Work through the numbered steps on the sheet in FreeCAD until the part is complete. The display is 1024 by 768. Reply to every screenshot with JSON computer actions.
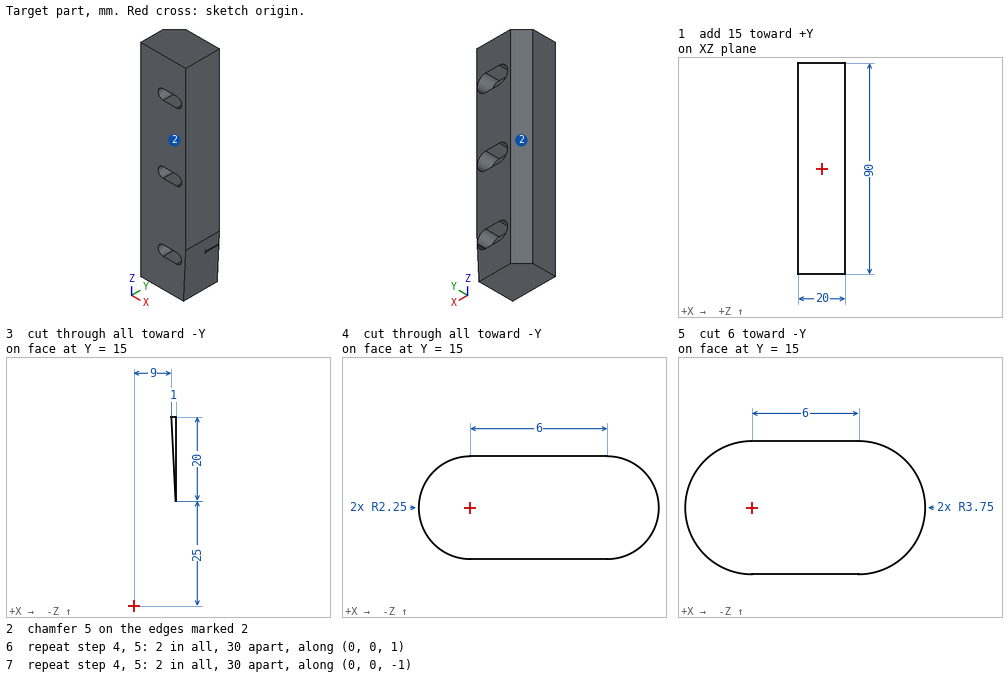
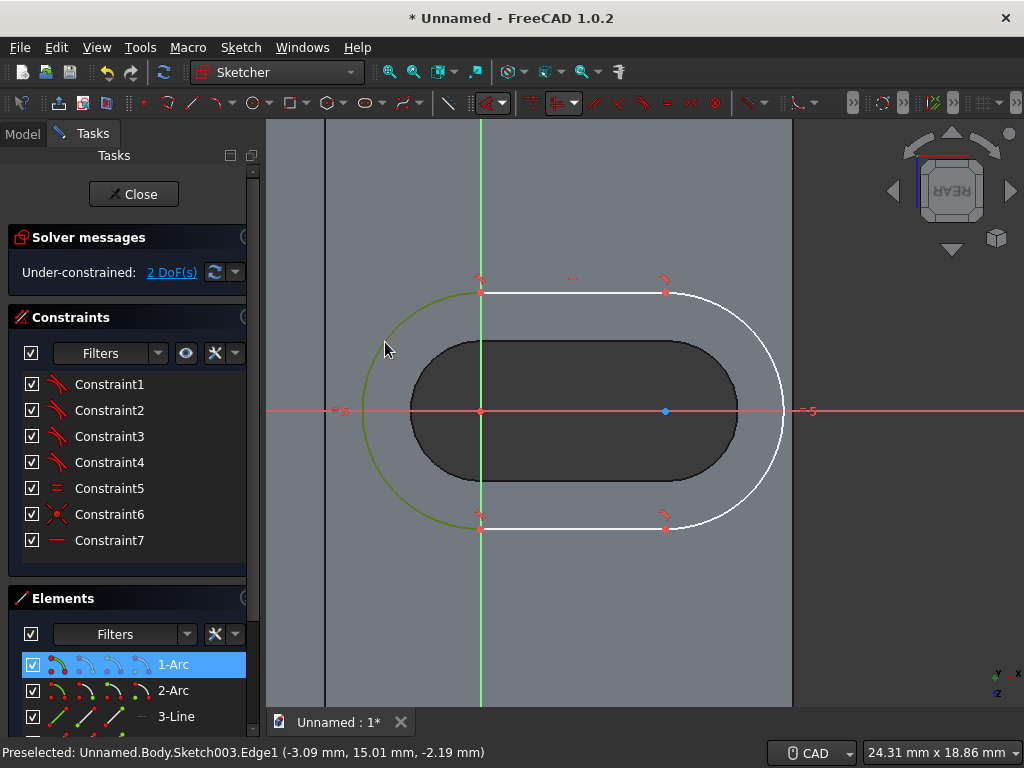
{"action": "left_click", "coordinate": [504, 104]}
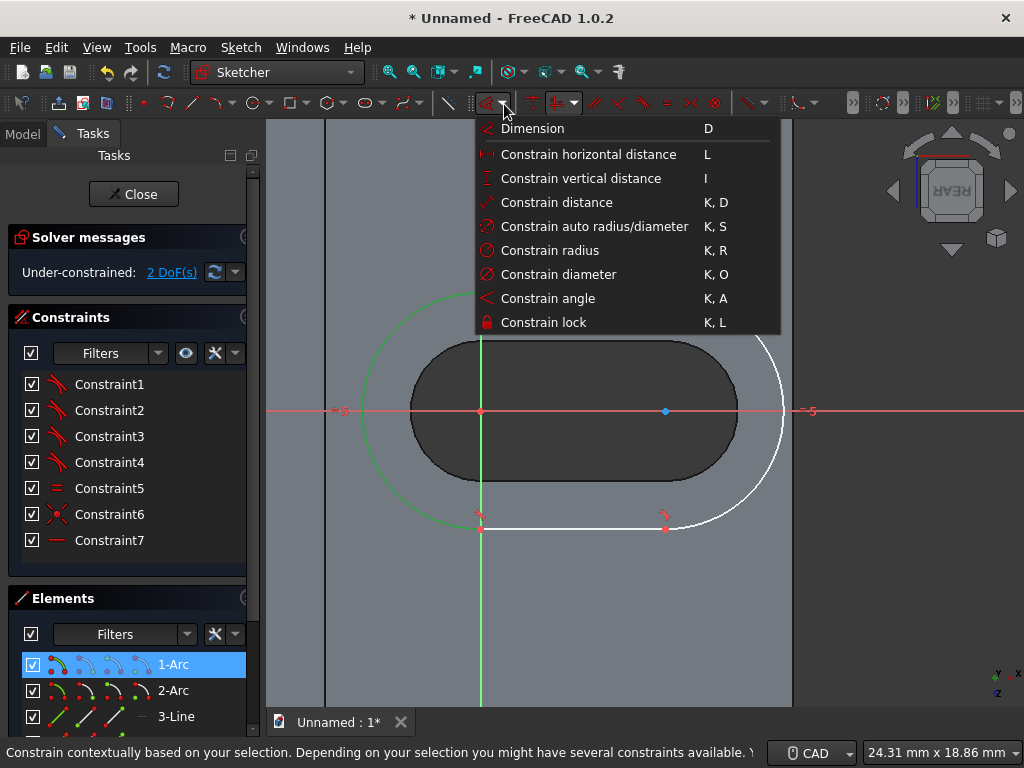
{"action": "left_click", "coordinate": [628, 250]}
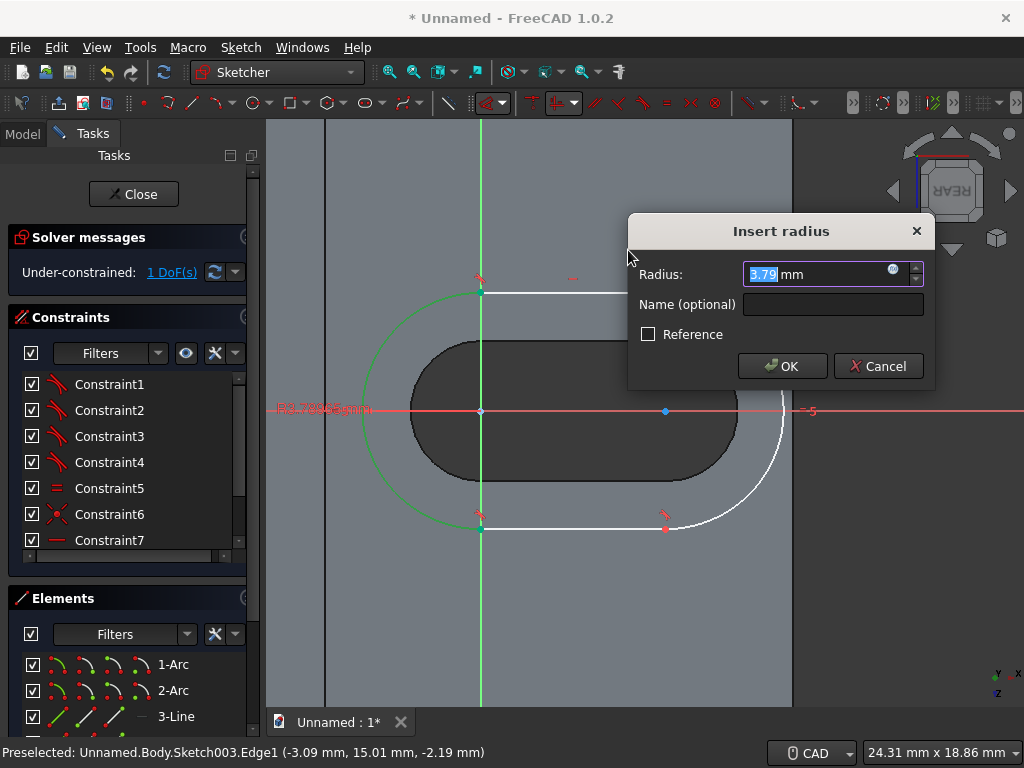
{"action": "type", "text": "3.75"}
{"action": "key", "text": "Return"}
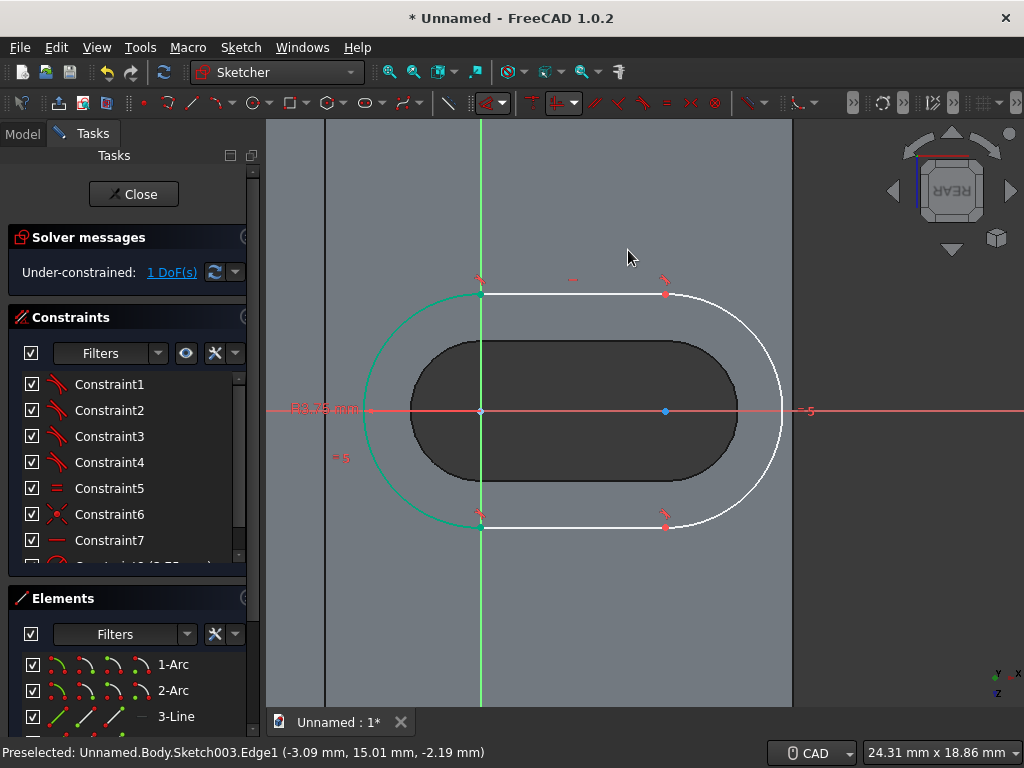
{"action": "left_click", "coordinate": [536, 294]}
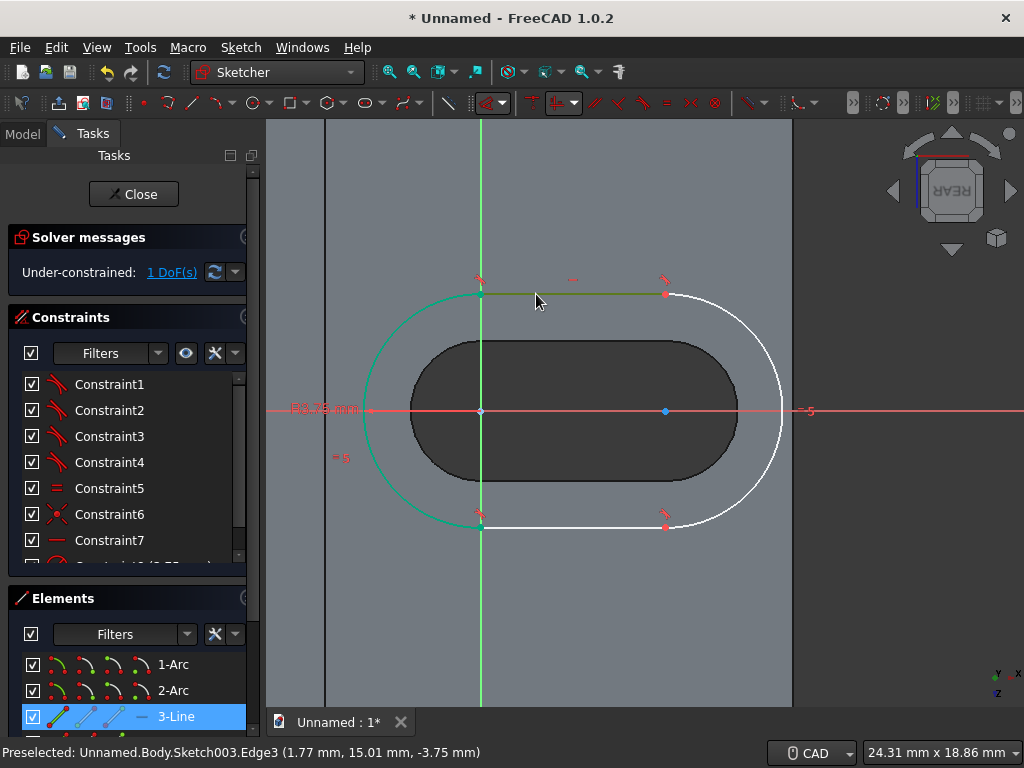
{"action": "left_click", "coordinate": [504, 104]}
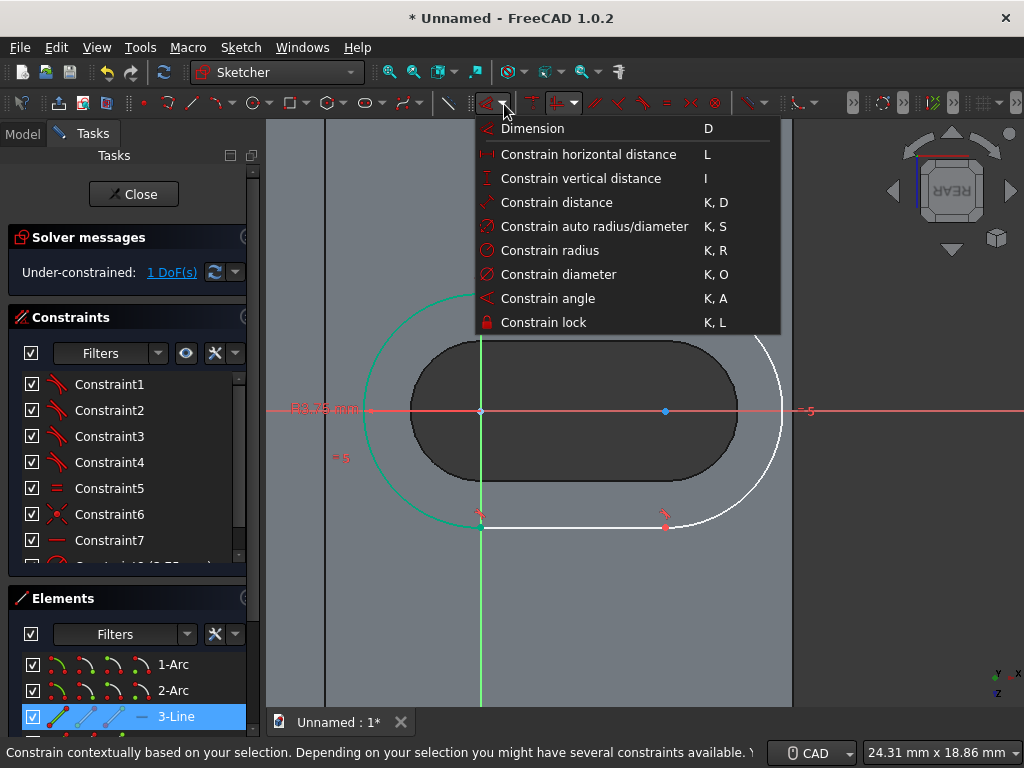
{"action": "left_click", "coordinate": [628, 154]}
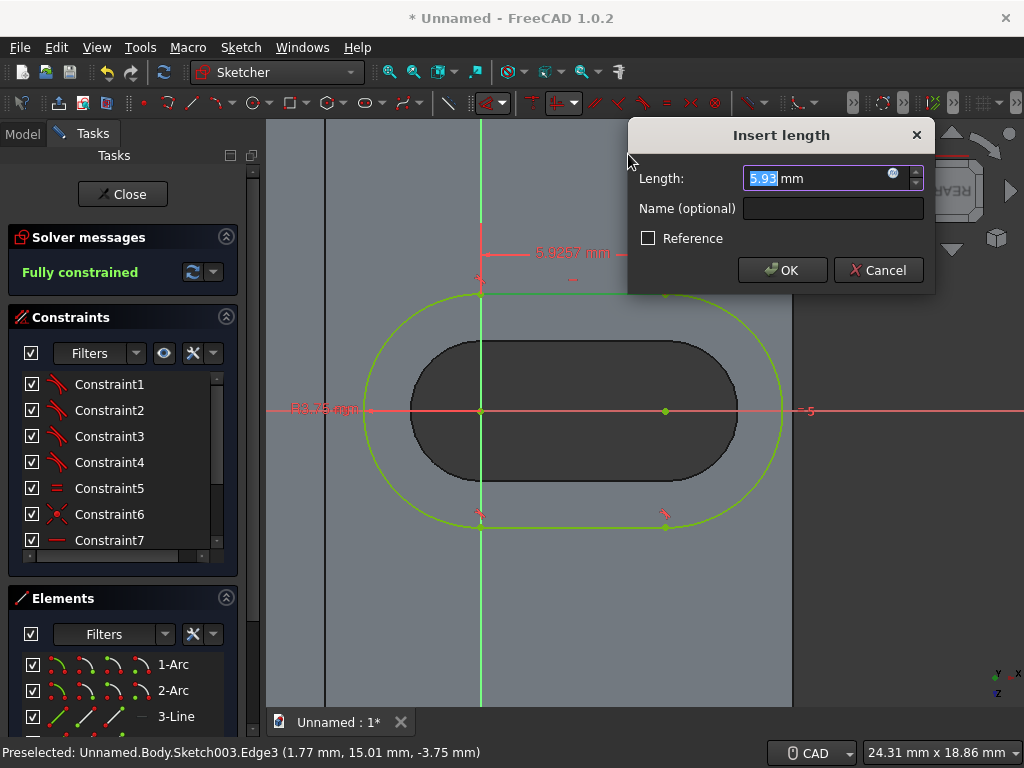
{"action": "type", "text": "6"}
{"action": "key", "text": "Return"}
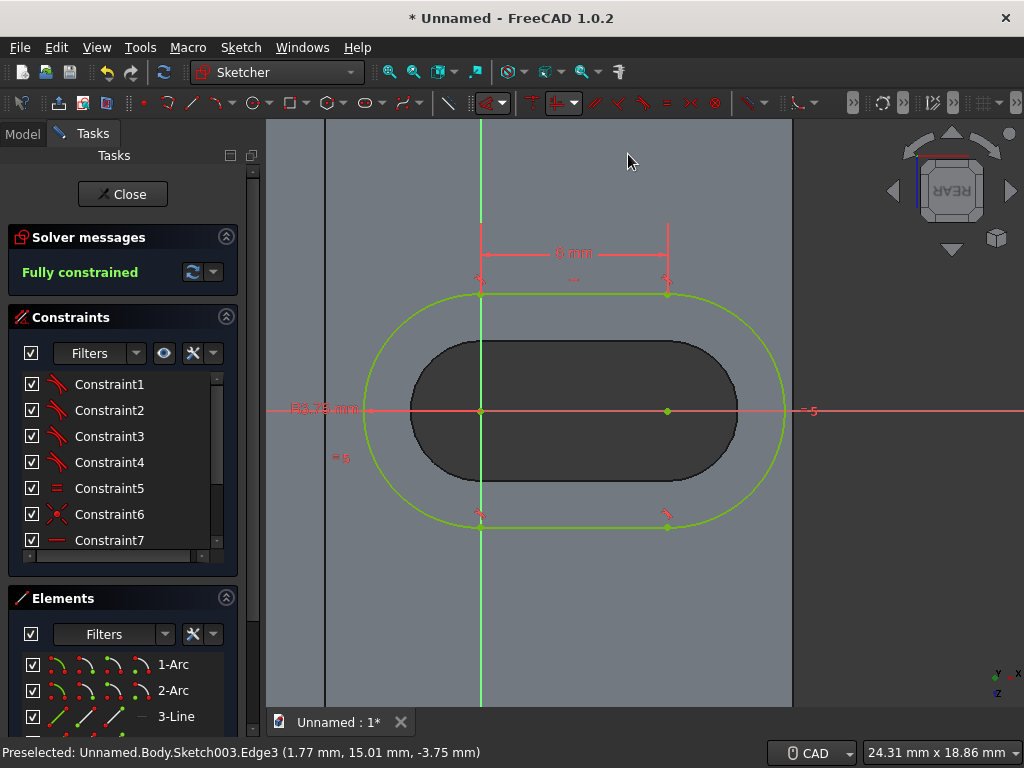
{"action": "left_click", "coordinate": [123, 194]}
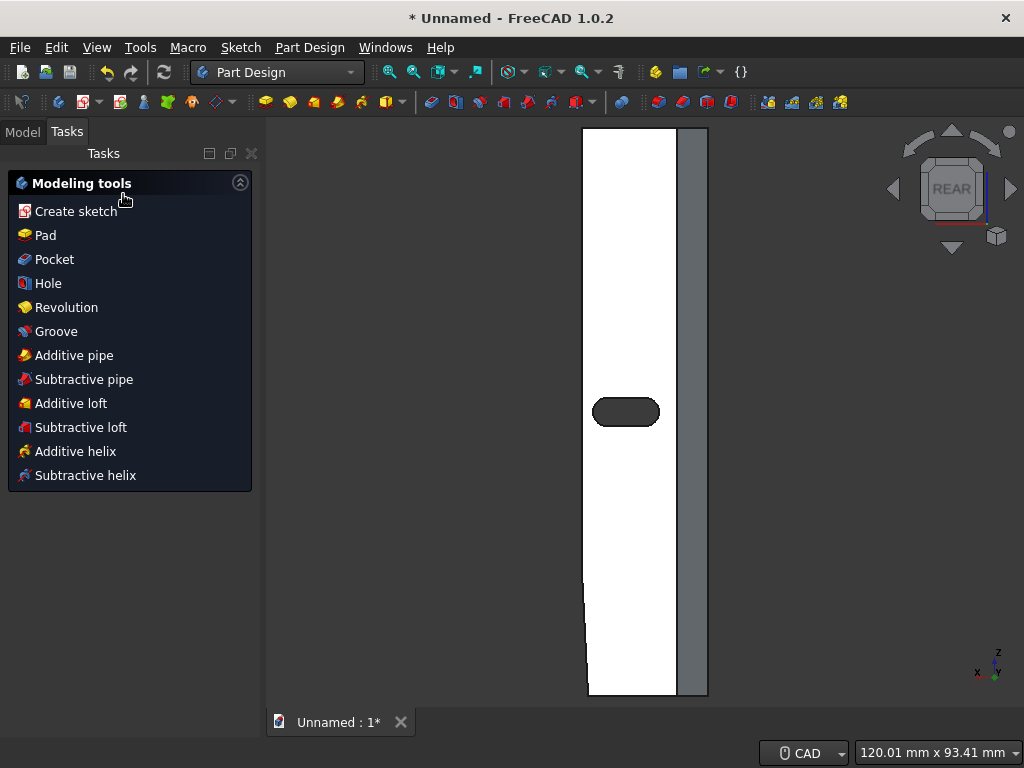
{"action": "left_click", "coordinate": [432, 102]}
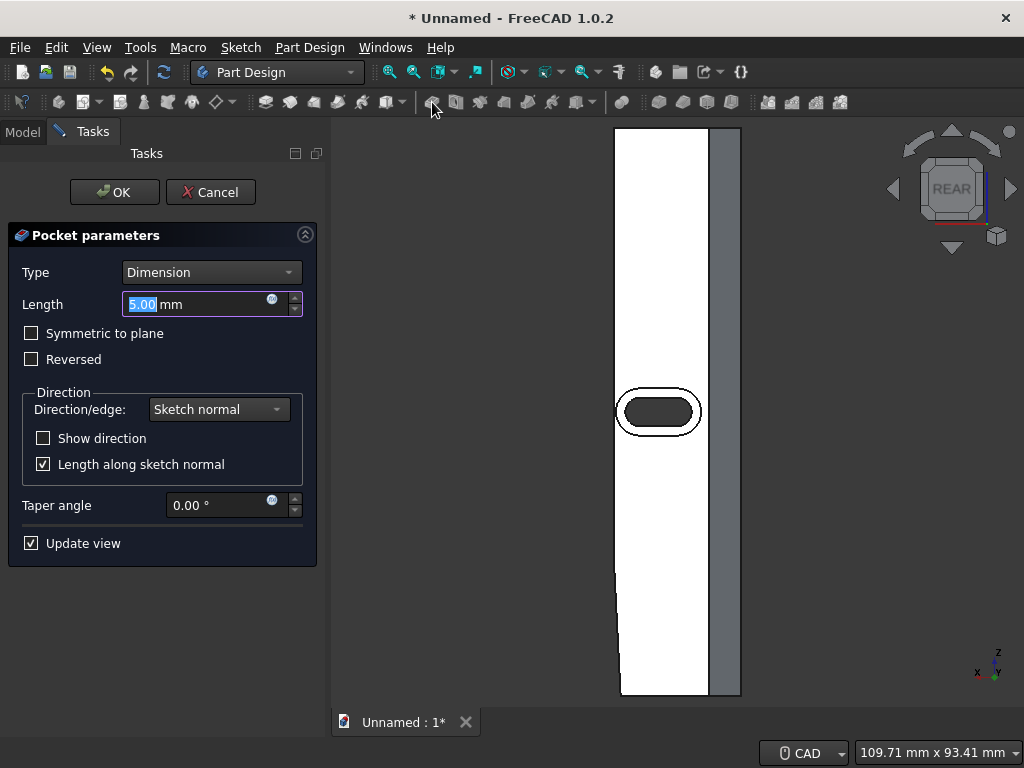
{"action": "type", "text": "6"}
{"action": "key", "text": "Tab"}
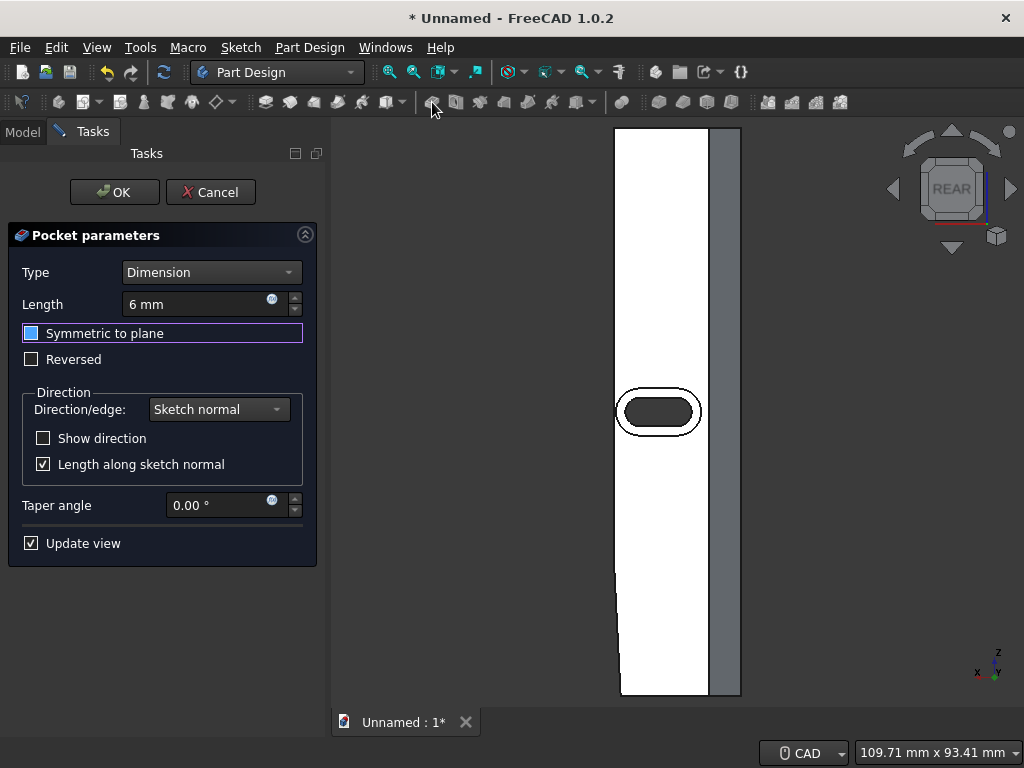
{"action": "left_click", "coordinate": [115, 192]}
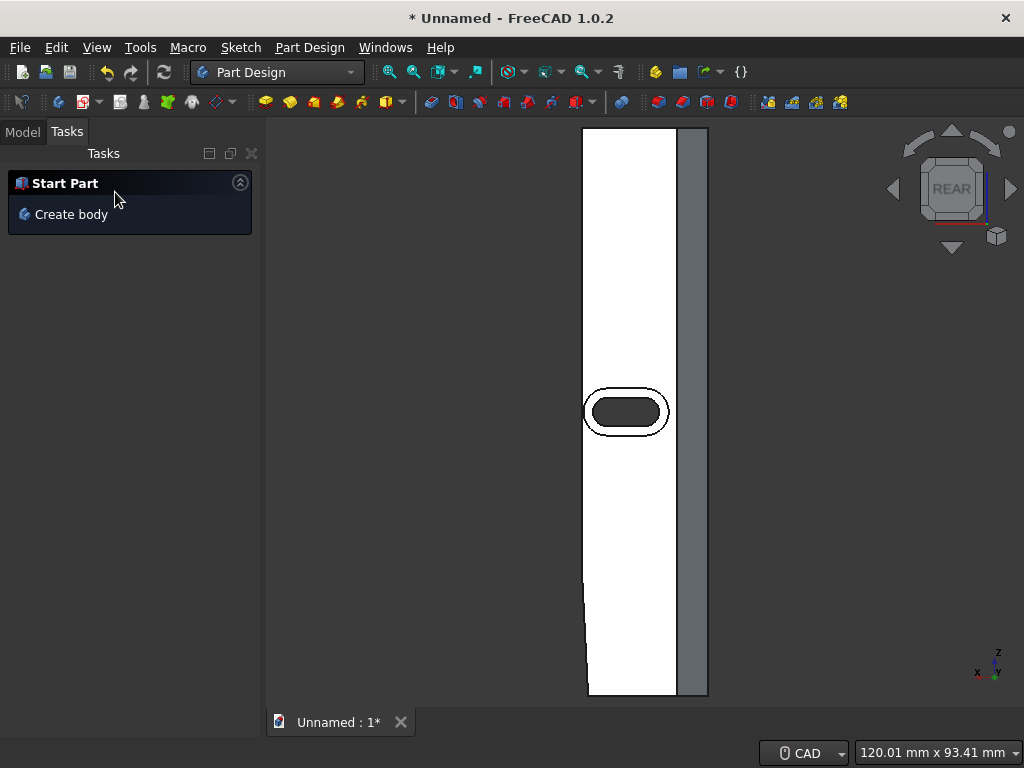
{"action": "left_click", "coordinate": [23, 131]}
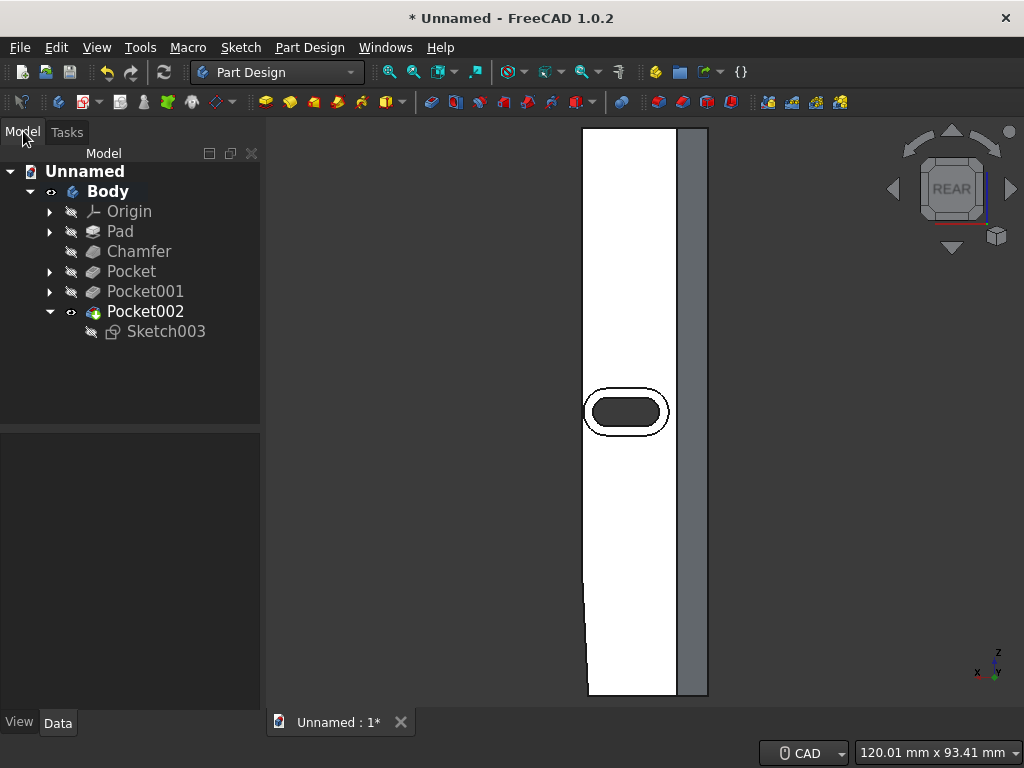
{"action": "left_click", "coordinate": [116, 292]}